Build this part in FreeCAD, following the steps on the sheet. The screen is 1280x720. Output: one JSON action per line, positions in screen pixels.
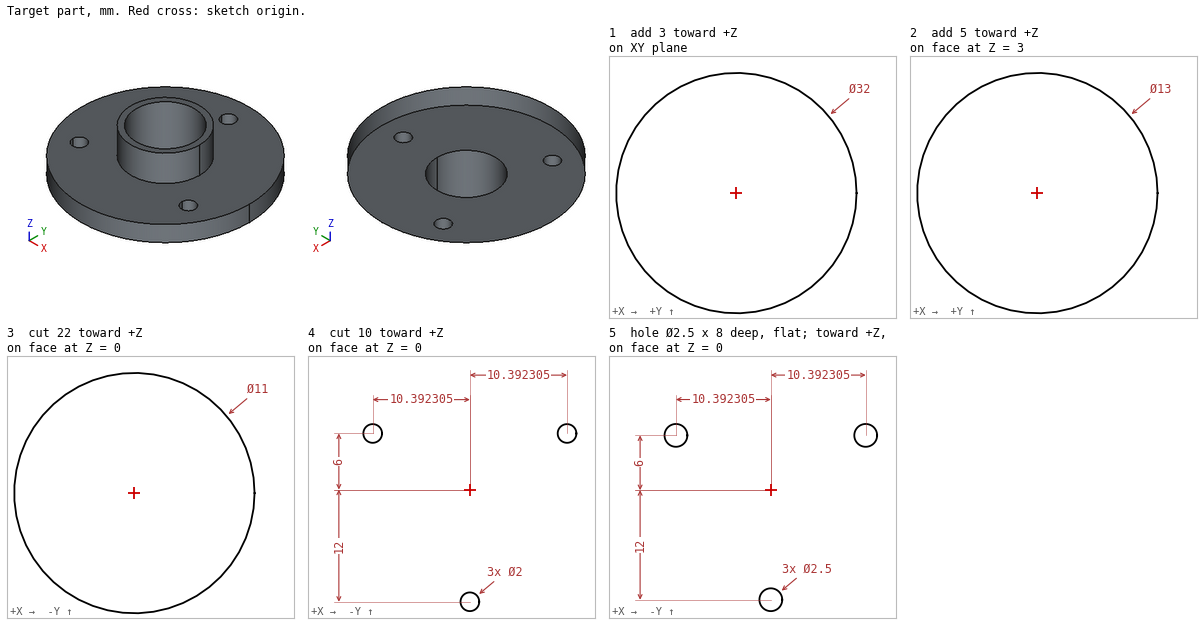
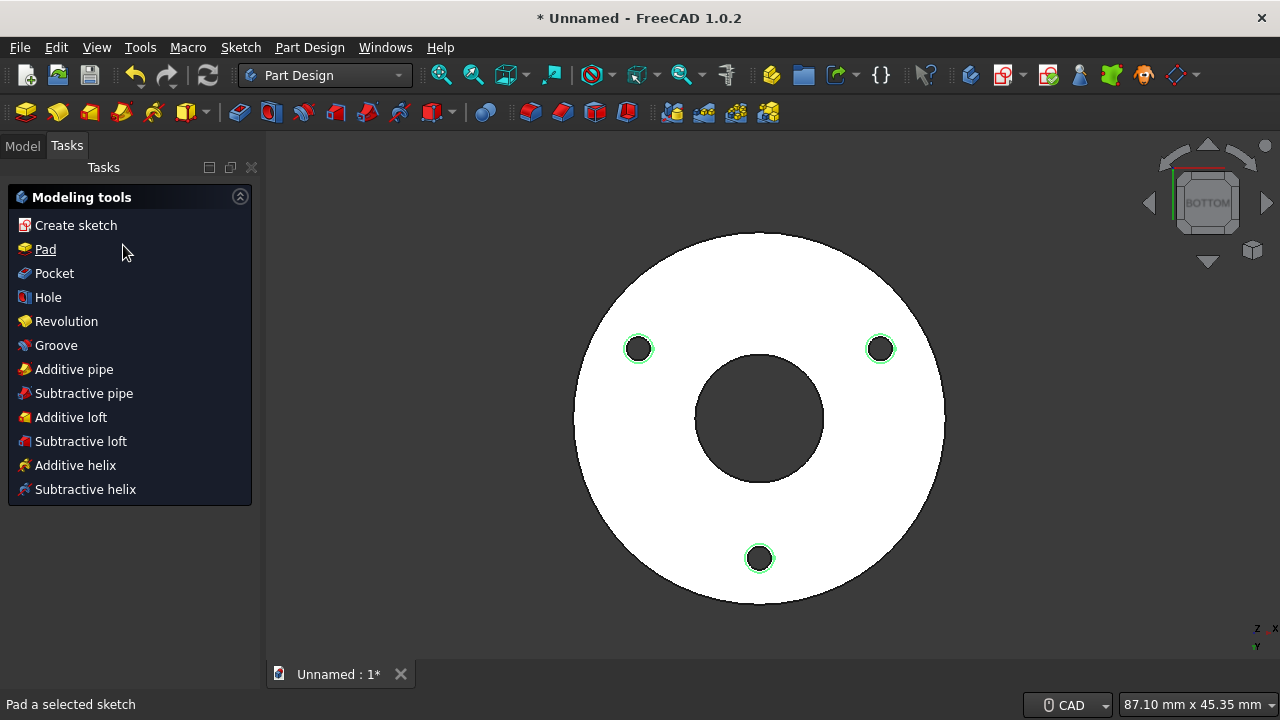
{"action": "left_click", "coordinate": [272, 112]}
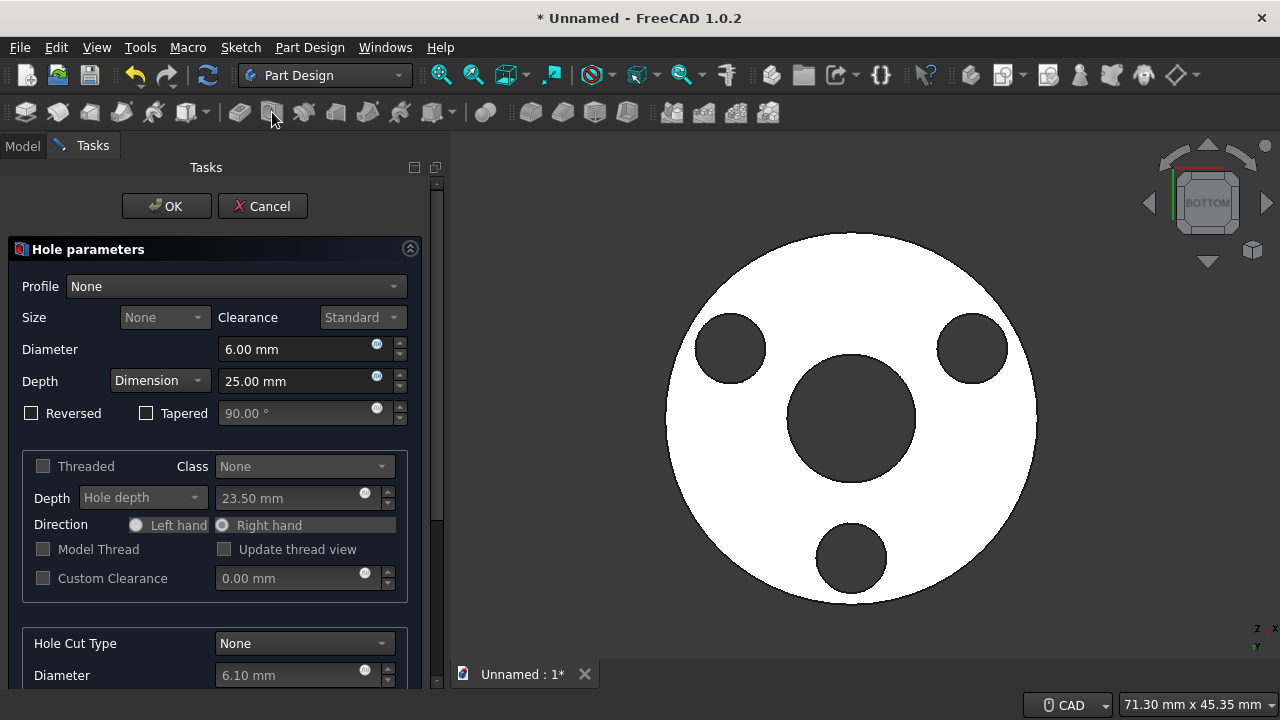
{"action": "triple_click", "coordinate": [305, 349]}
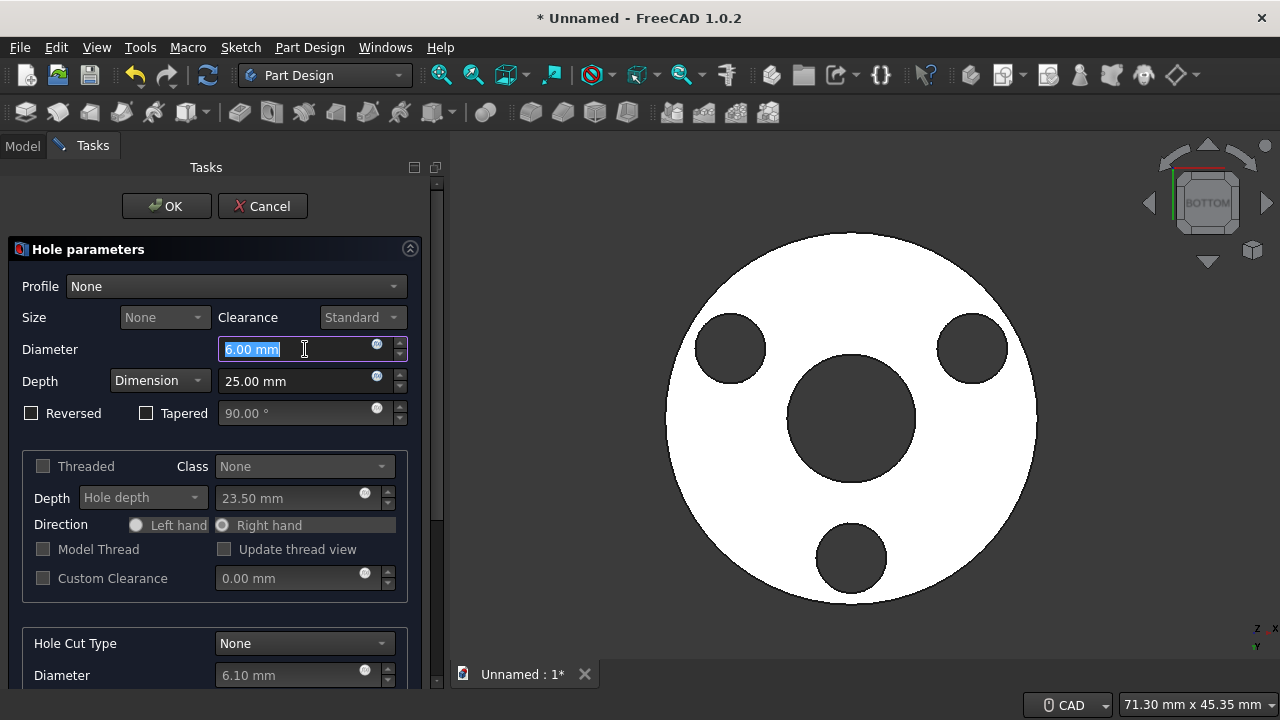
{"action": "type", "text": "2.5"}
{"action": "key", "text": "Tab"}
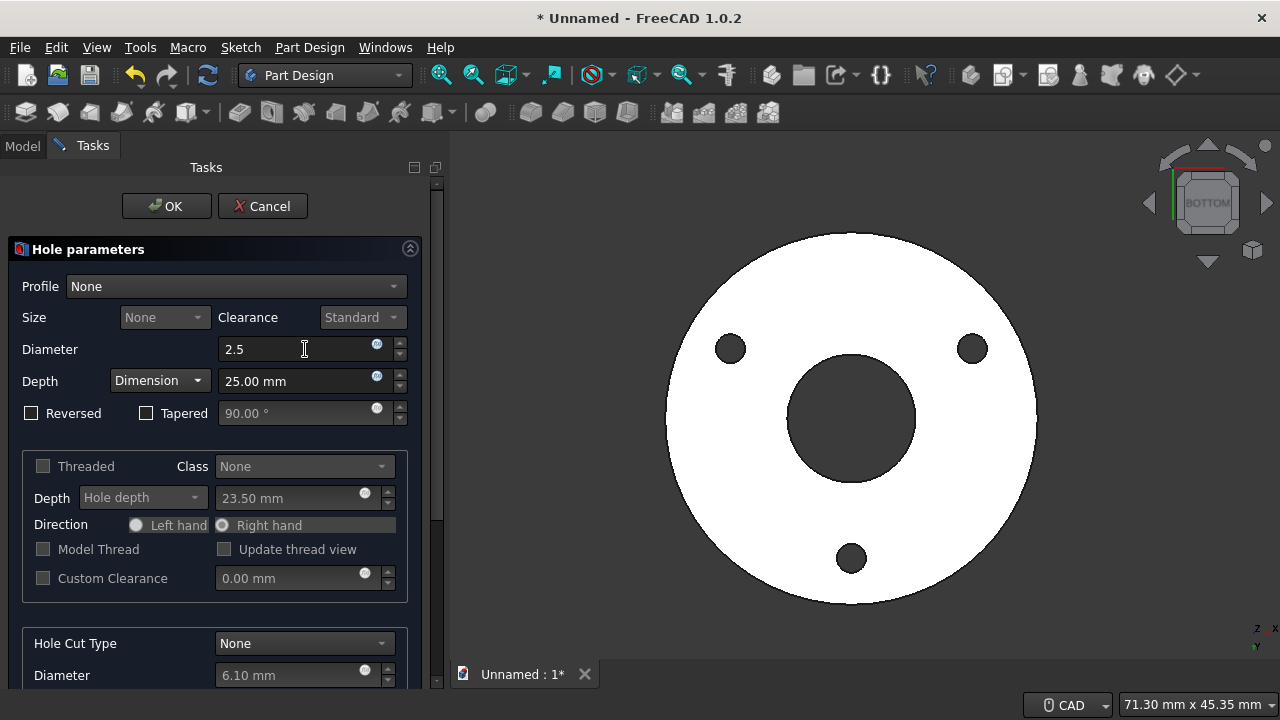
{"action": "triple_click", "coordinate": [305, 381]}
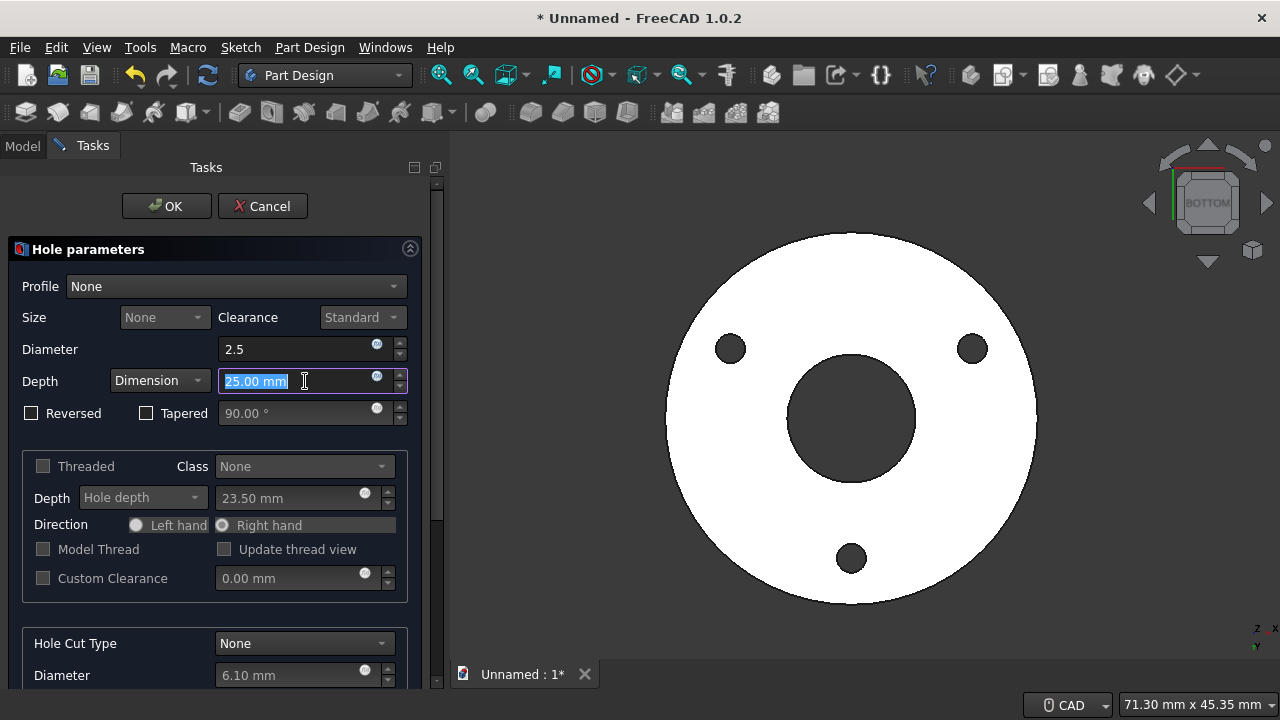
{"action": "type", "text": "8"}
{"action": "key", "text": "Tab"}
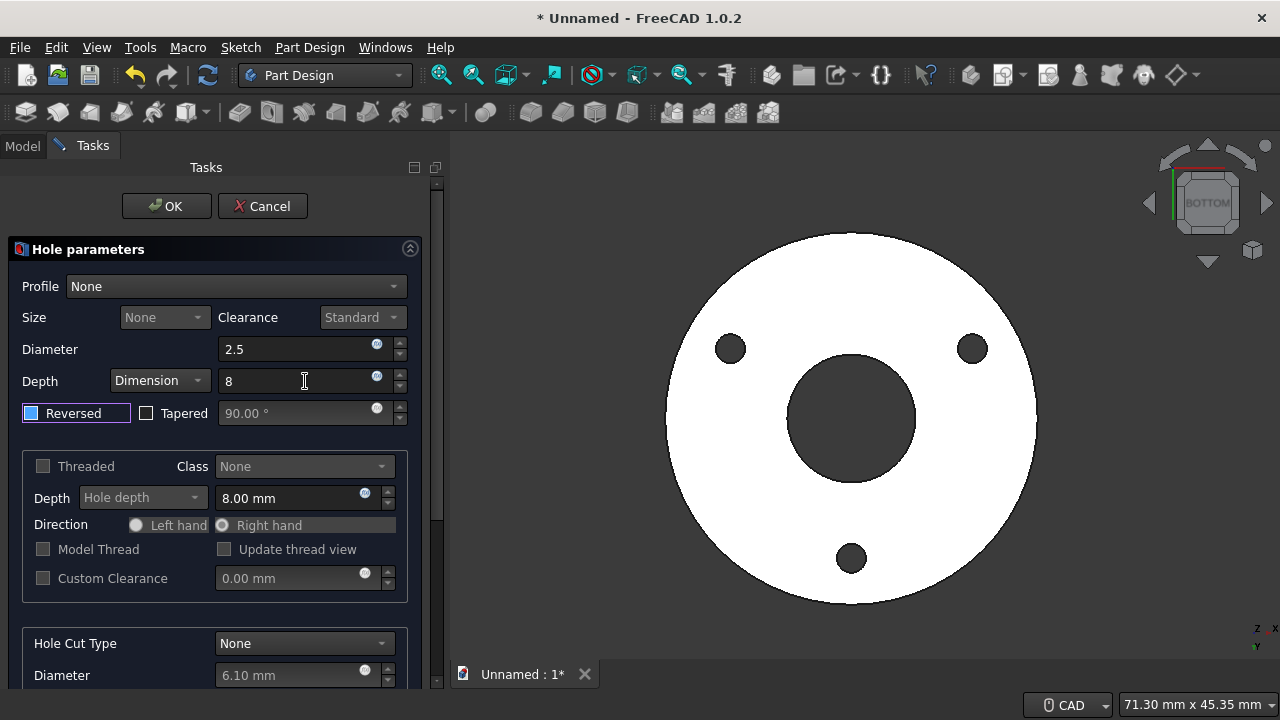
{"action": "scroll", "coordinate": [437, 432], "scroll_direction": "down", "scroll_amount": 4}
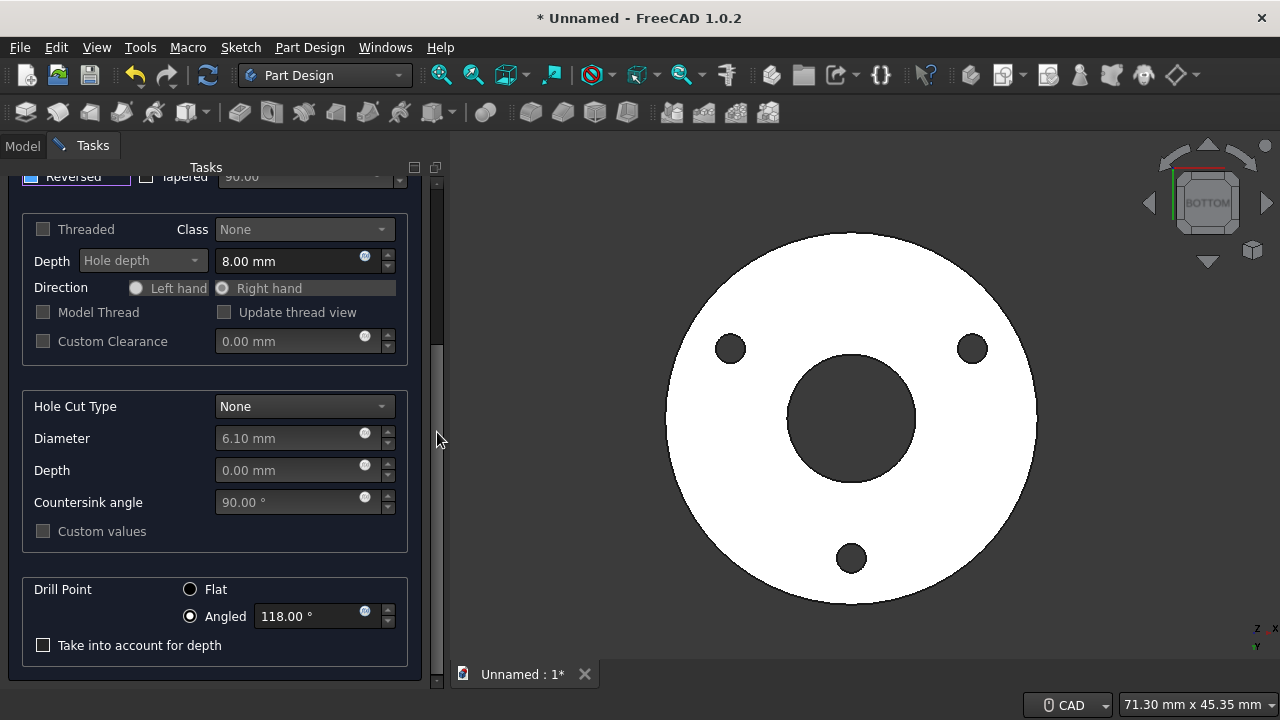
{"action": "left_click", "coordinate": [191, 589]}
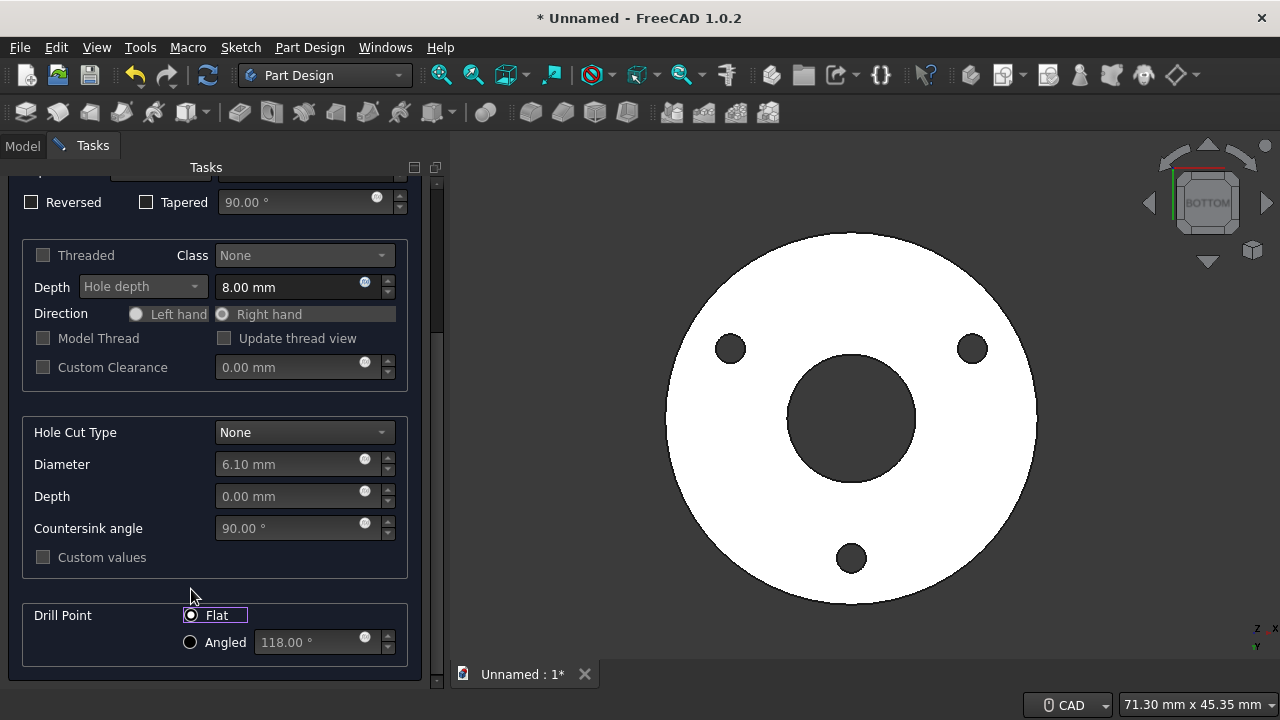
{"action": "scroll", "coordinate": [437, 432], "scroll_direction": "up", "scroll_amount": 5}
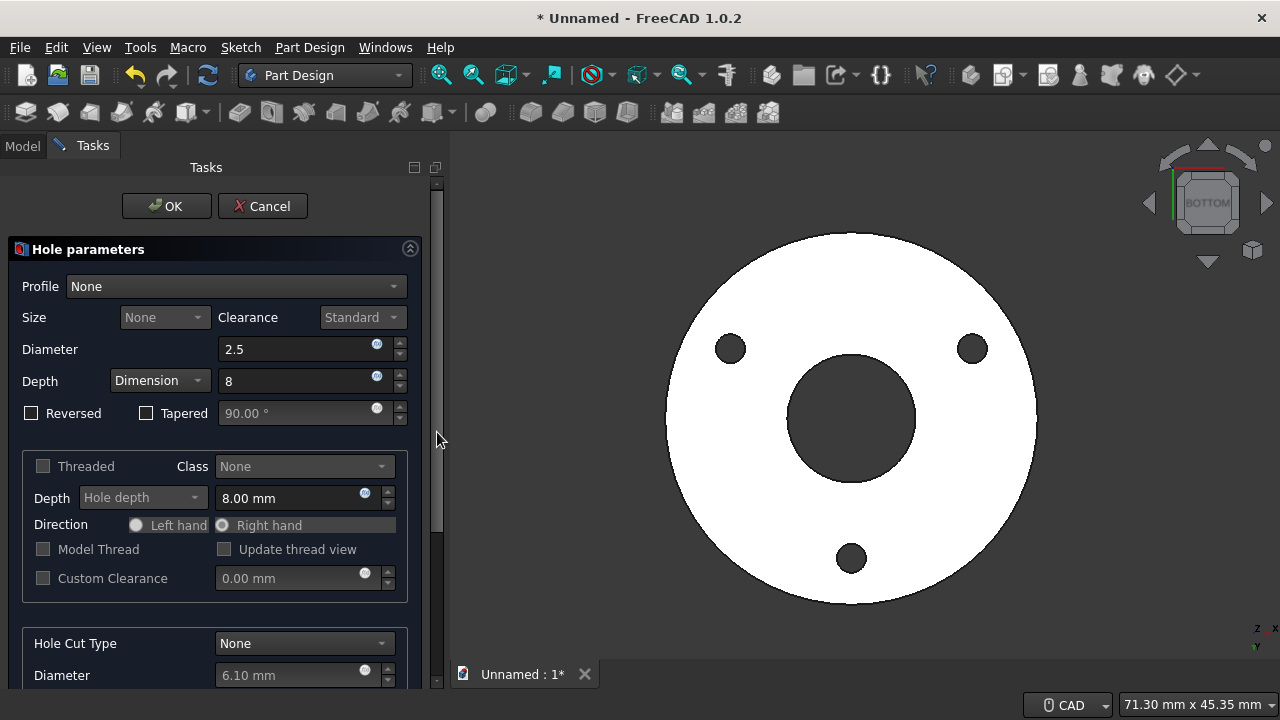
{"action": "left_click", "coordinate": [167, 206]}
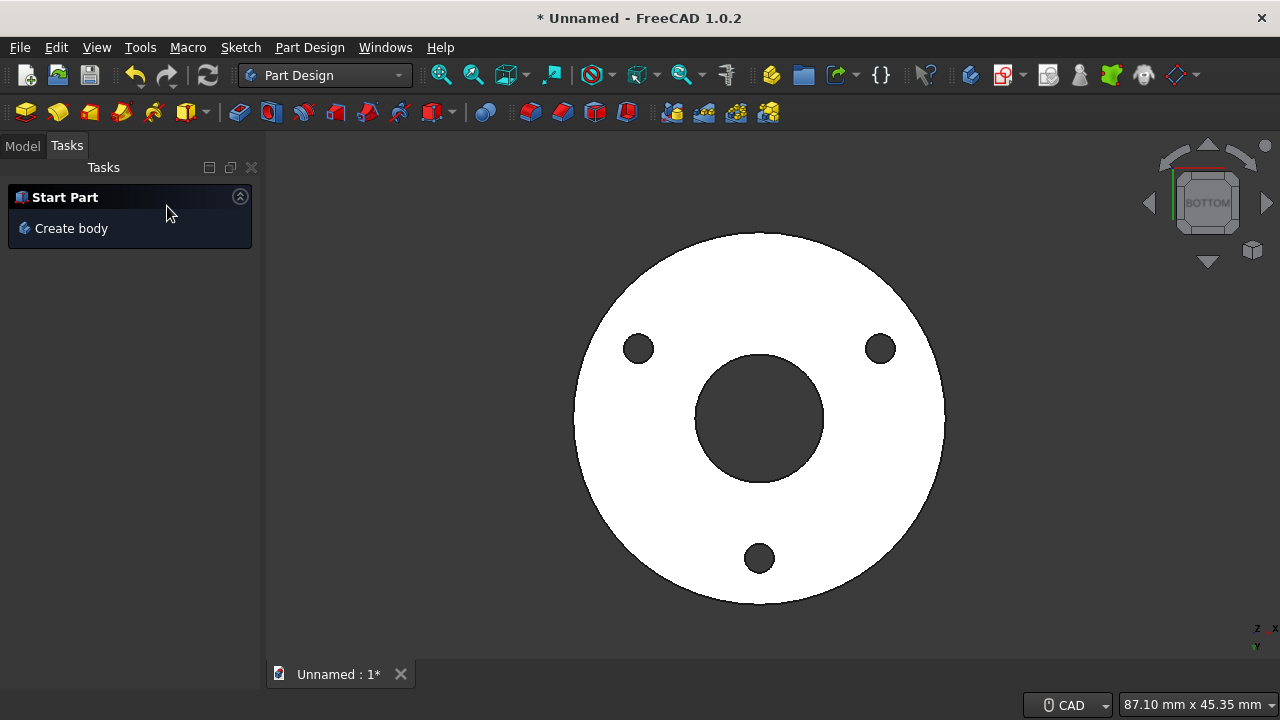
{"action": "key", "text": "0"}